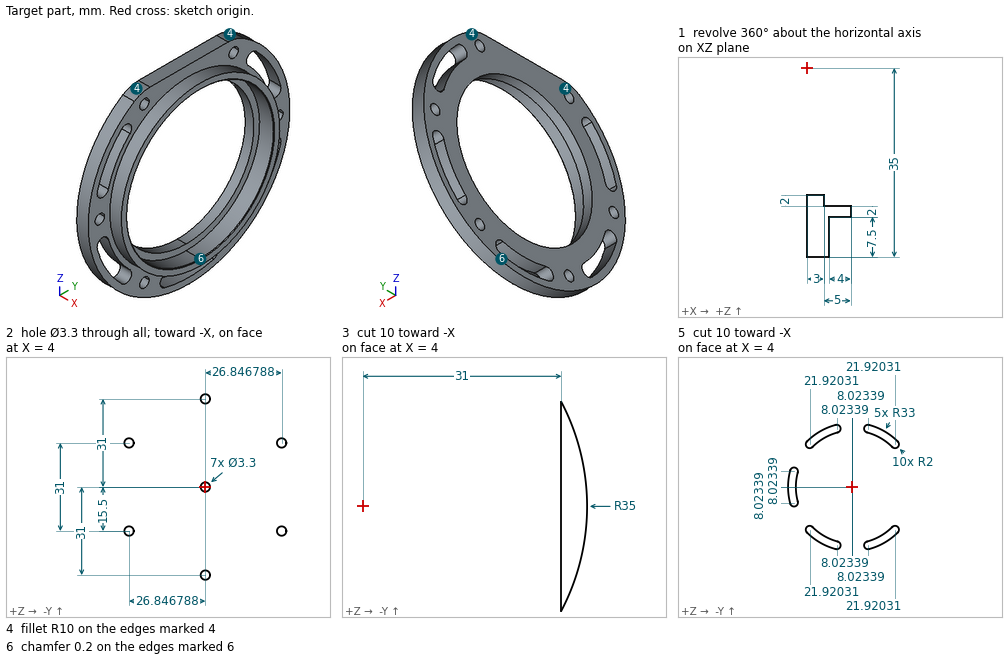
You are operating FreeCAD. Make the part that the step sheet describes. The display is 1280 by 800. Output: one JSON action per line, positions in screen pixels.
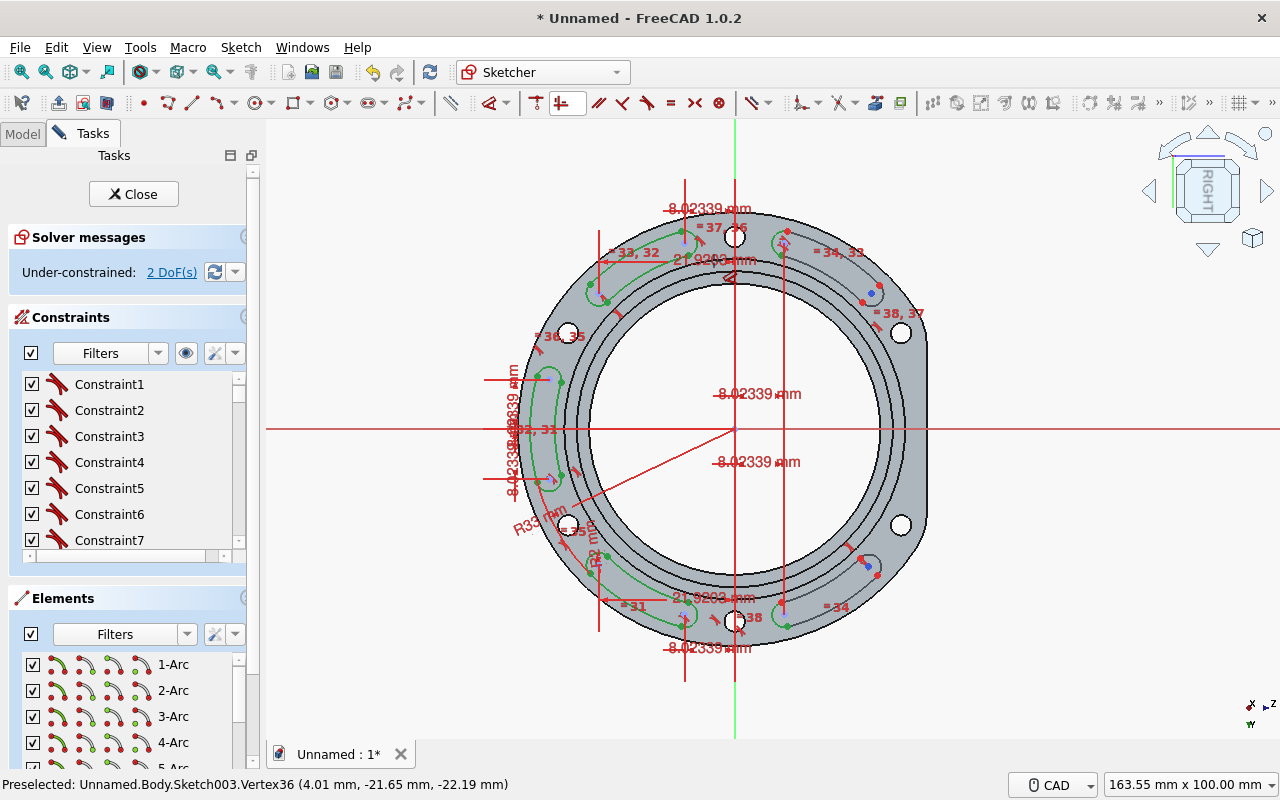
{"action": "left_click", "coordinate": [871, 294]}
{"action": "left_click", "coordinate": [834, 463]}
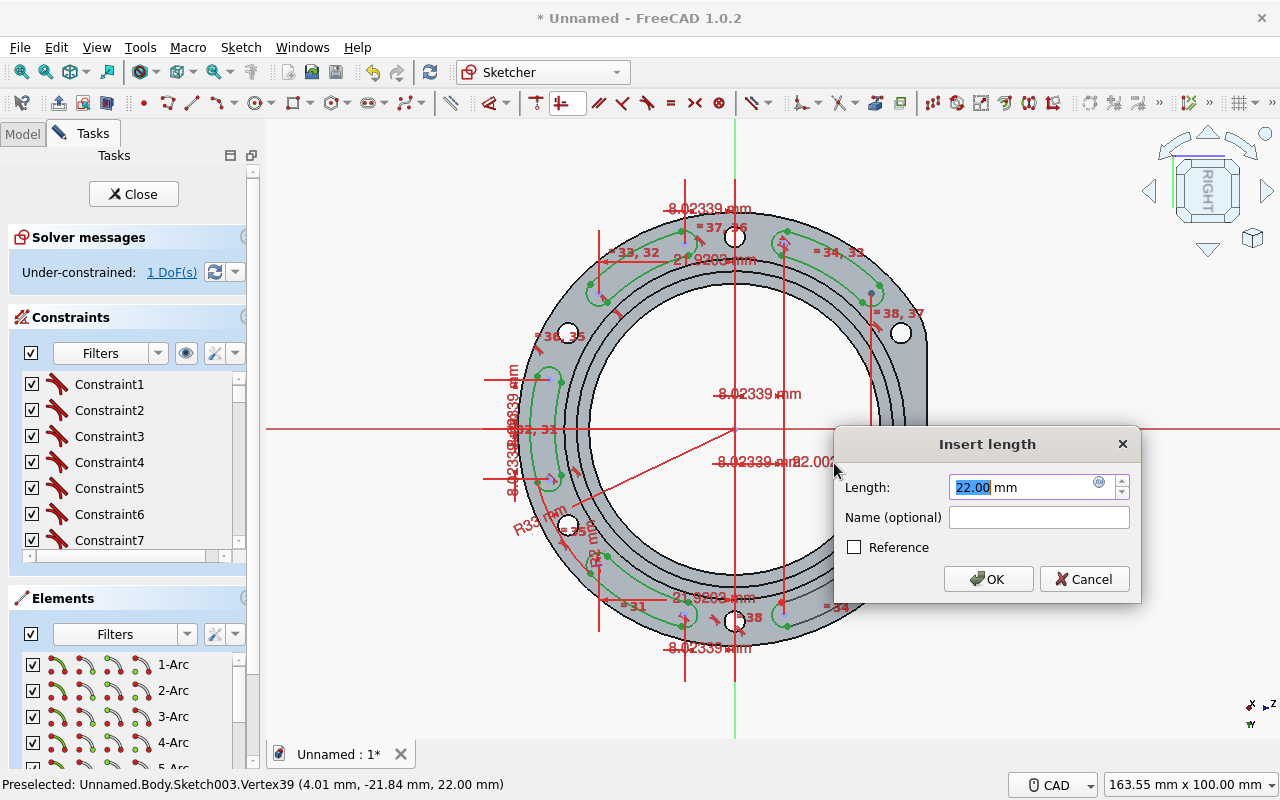
{"action": "type", "text": "21.92031"}
{"action": "key", "text": "Return"}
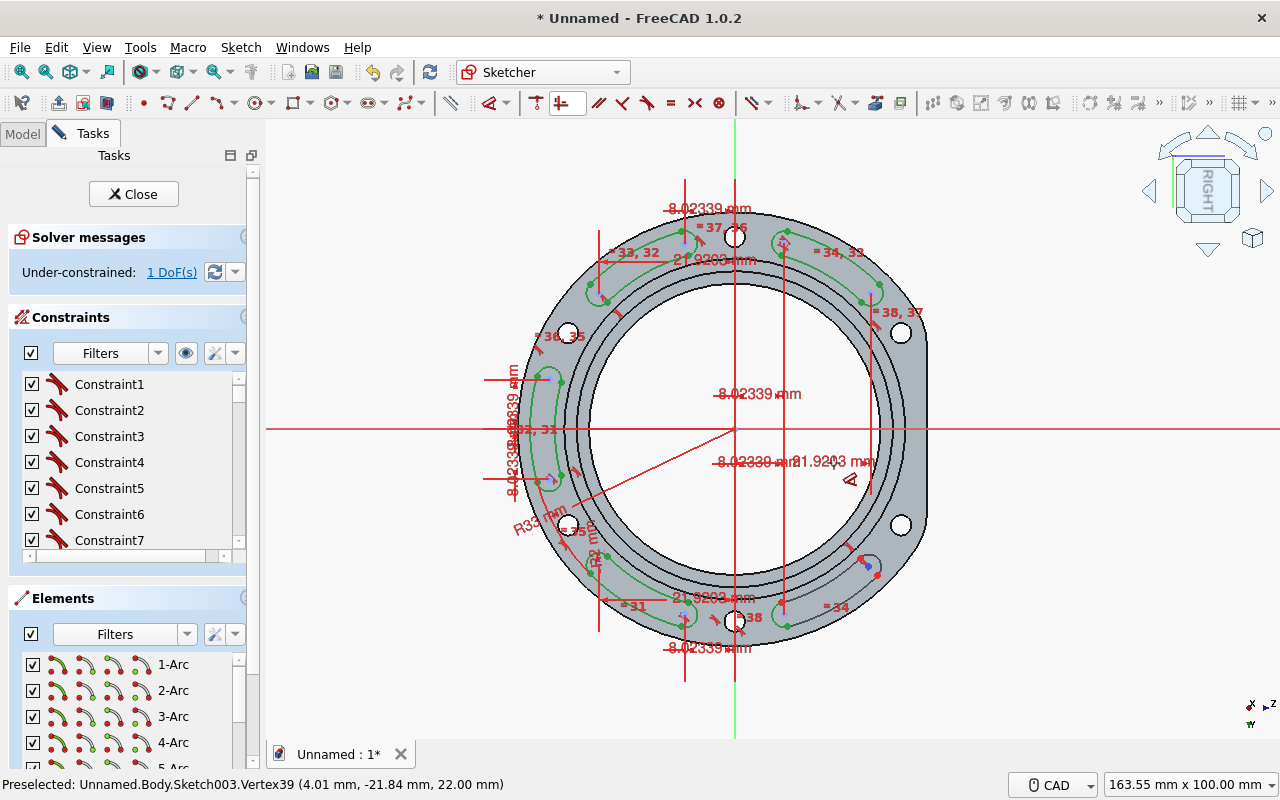
{"action": "left_click", "coordinate": [869, 567]}
{"action": "left_click", "coordinate": [833, 395]}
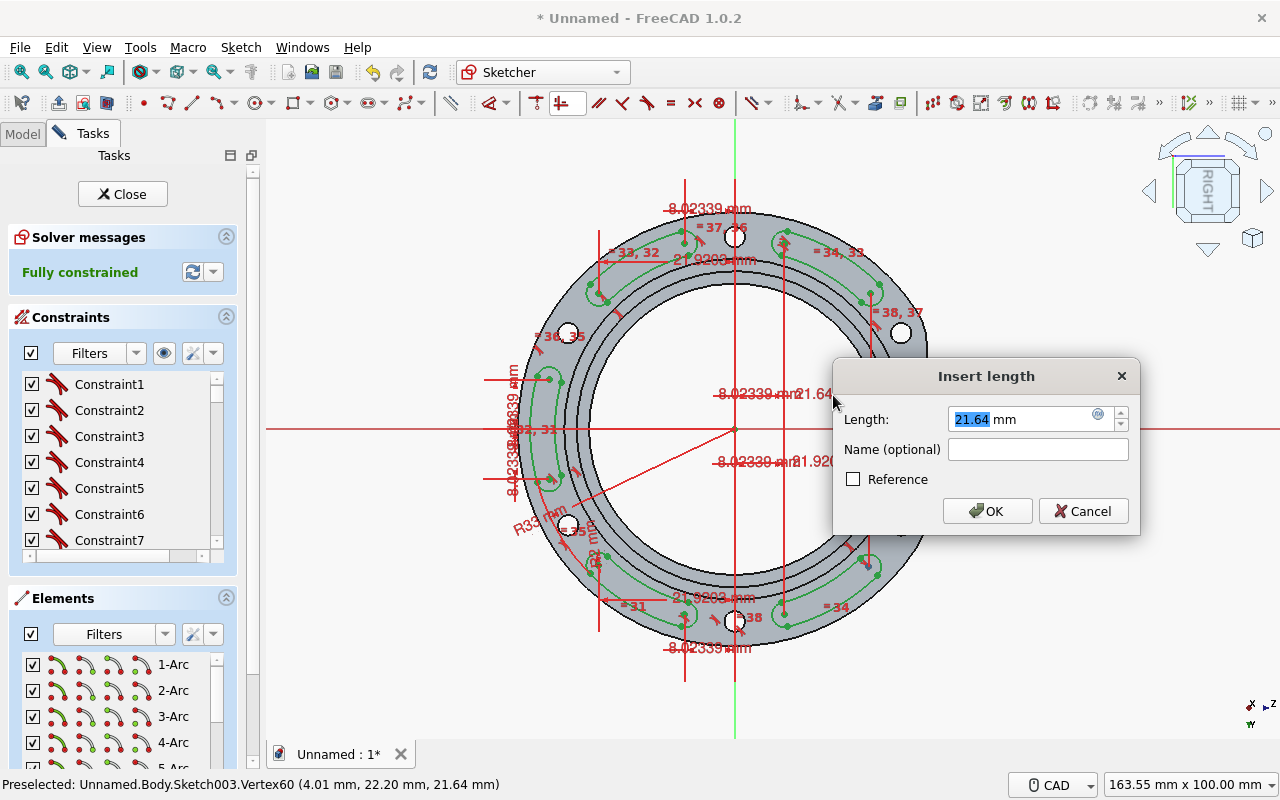
{"action": "type", "text": "21.92031"}
{"action": "key", "text": "Return"}
{"action": "key", "text": "Escape"}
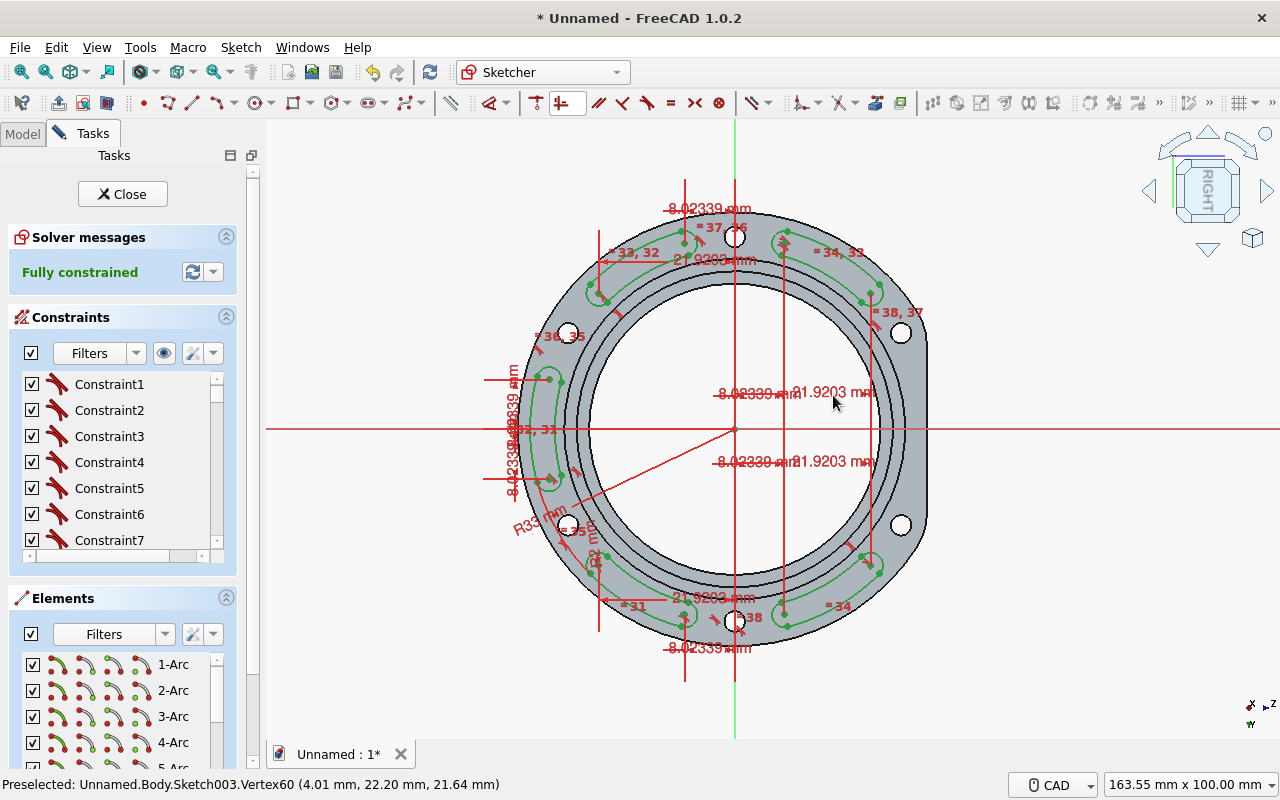
{"action": "left_click", "coordinate": [123, 194]}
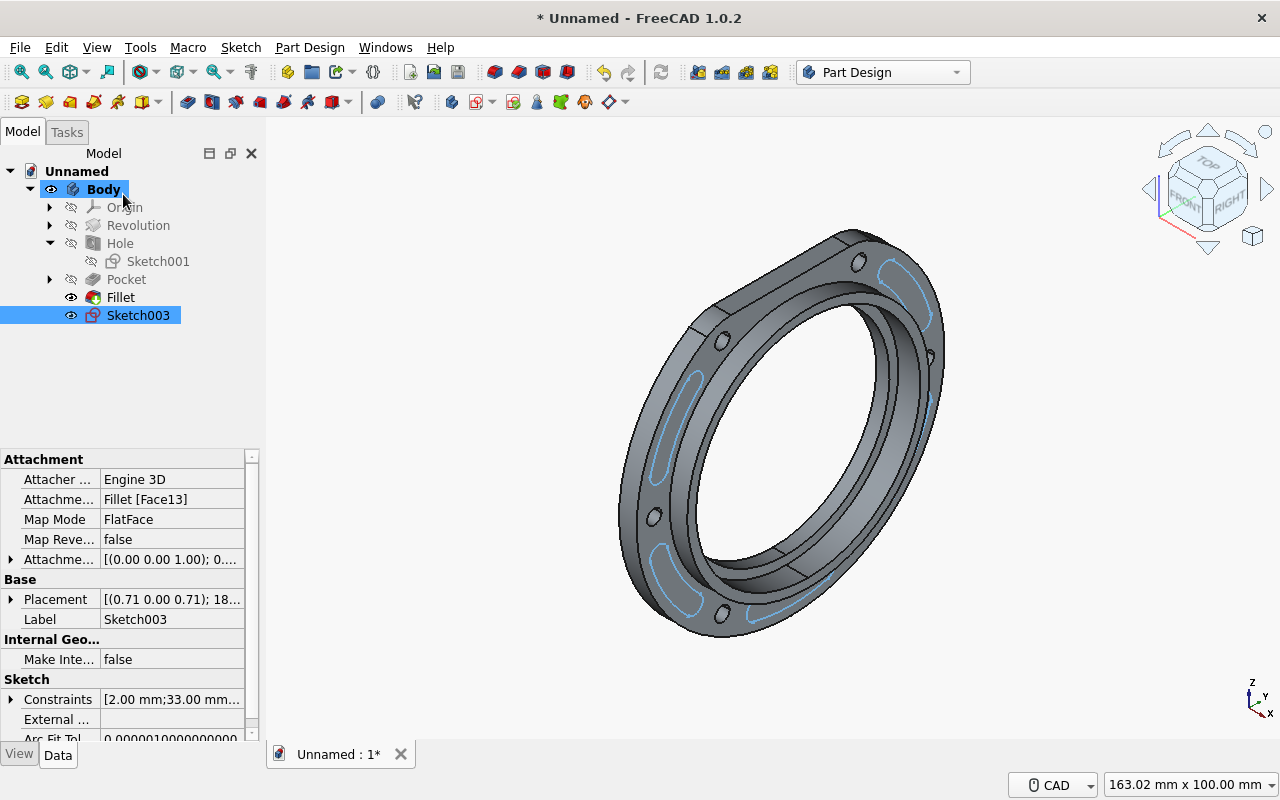
{"action": "left_click", "coordinate": [188, 102]}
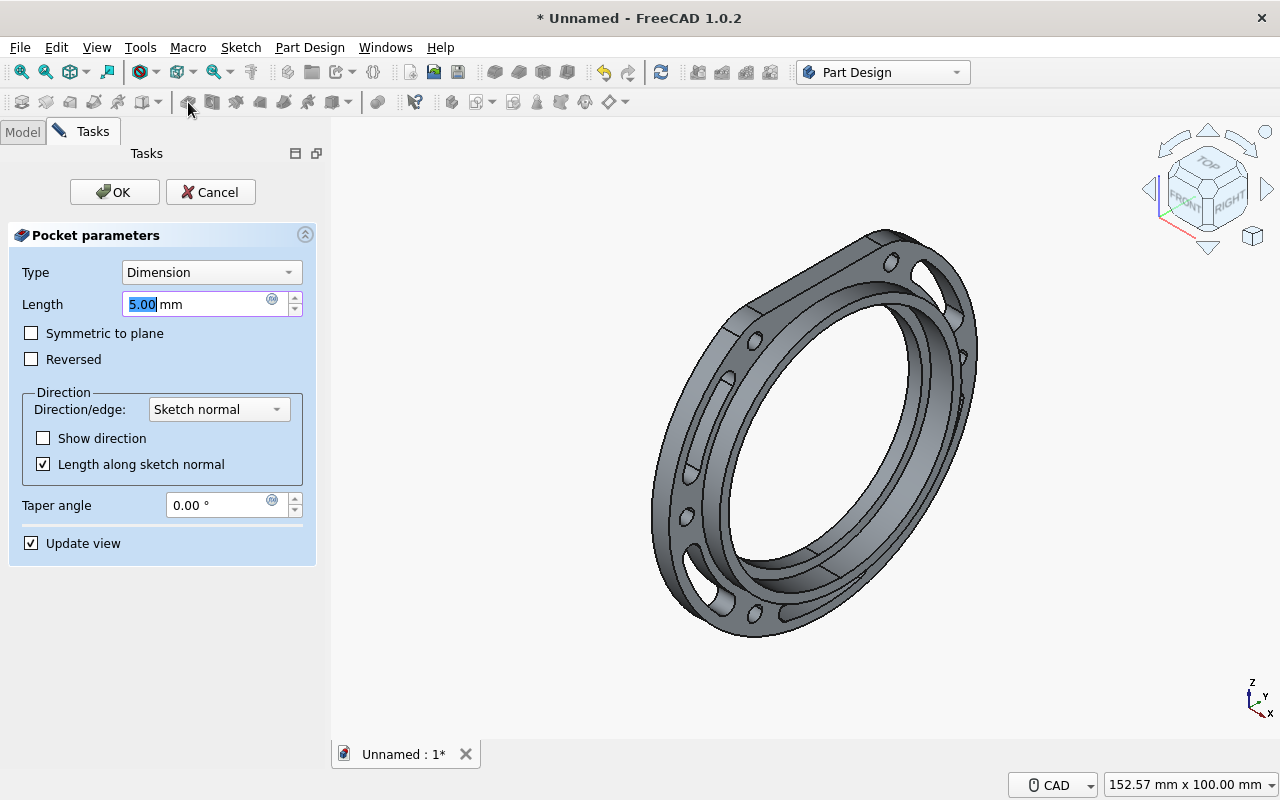
{"action": "type", "text": "10"}
{"action": "key", "text": "Tab"}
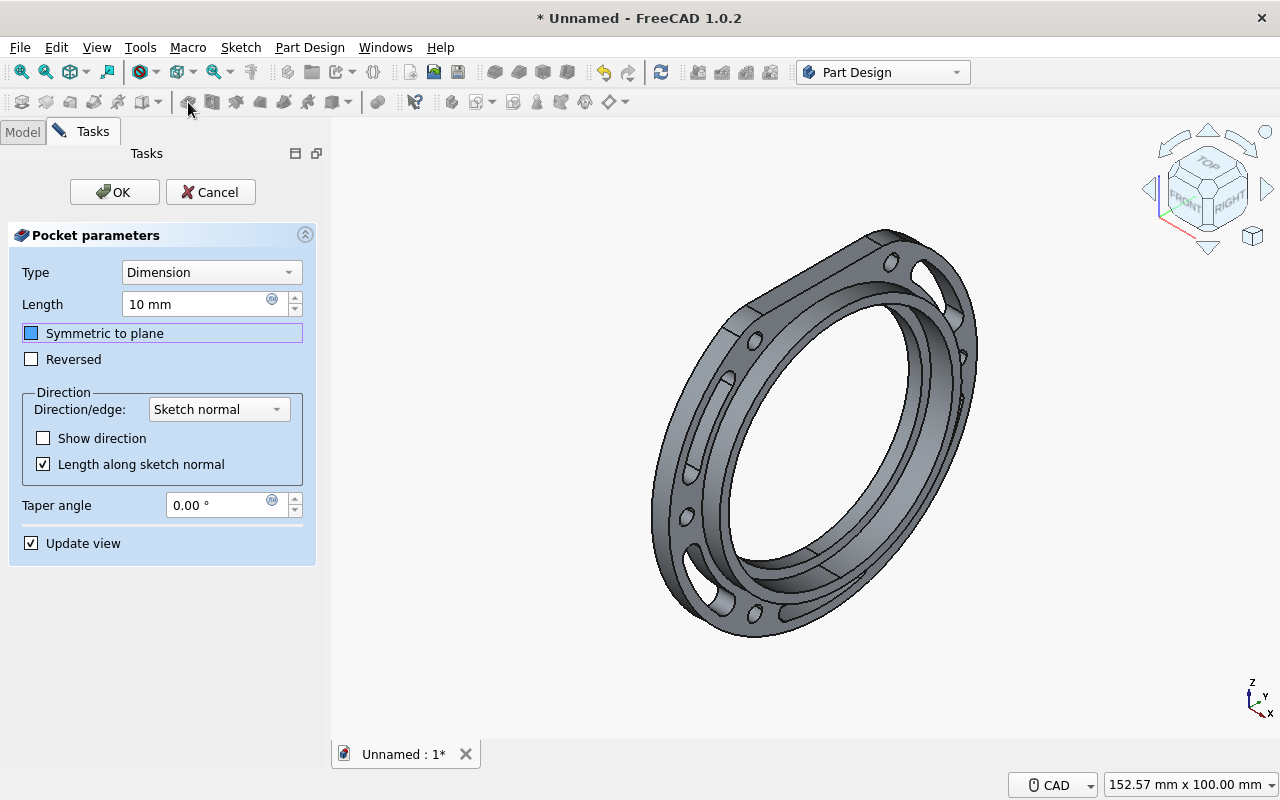
{"action": "left_click", "coordinate": [115, 192]}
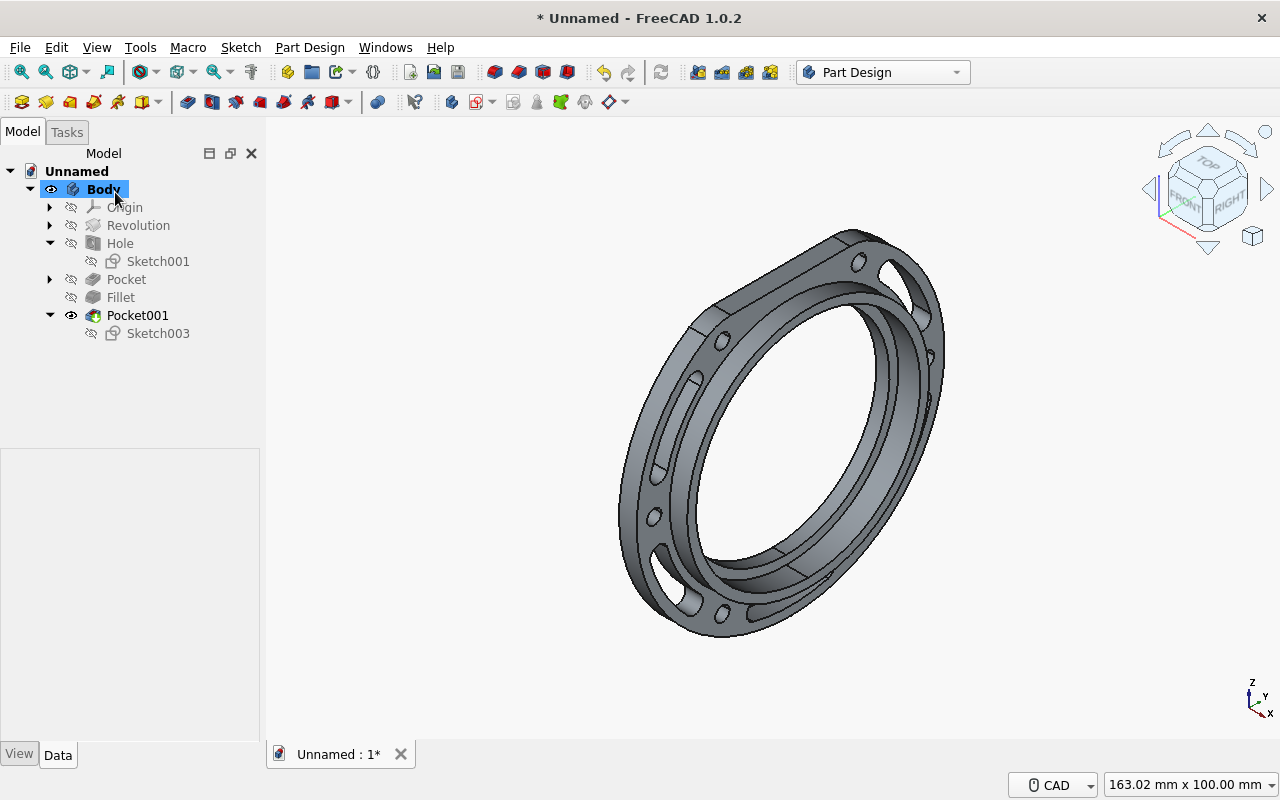
{"action": "left_click", "coordinate": [915, 346]}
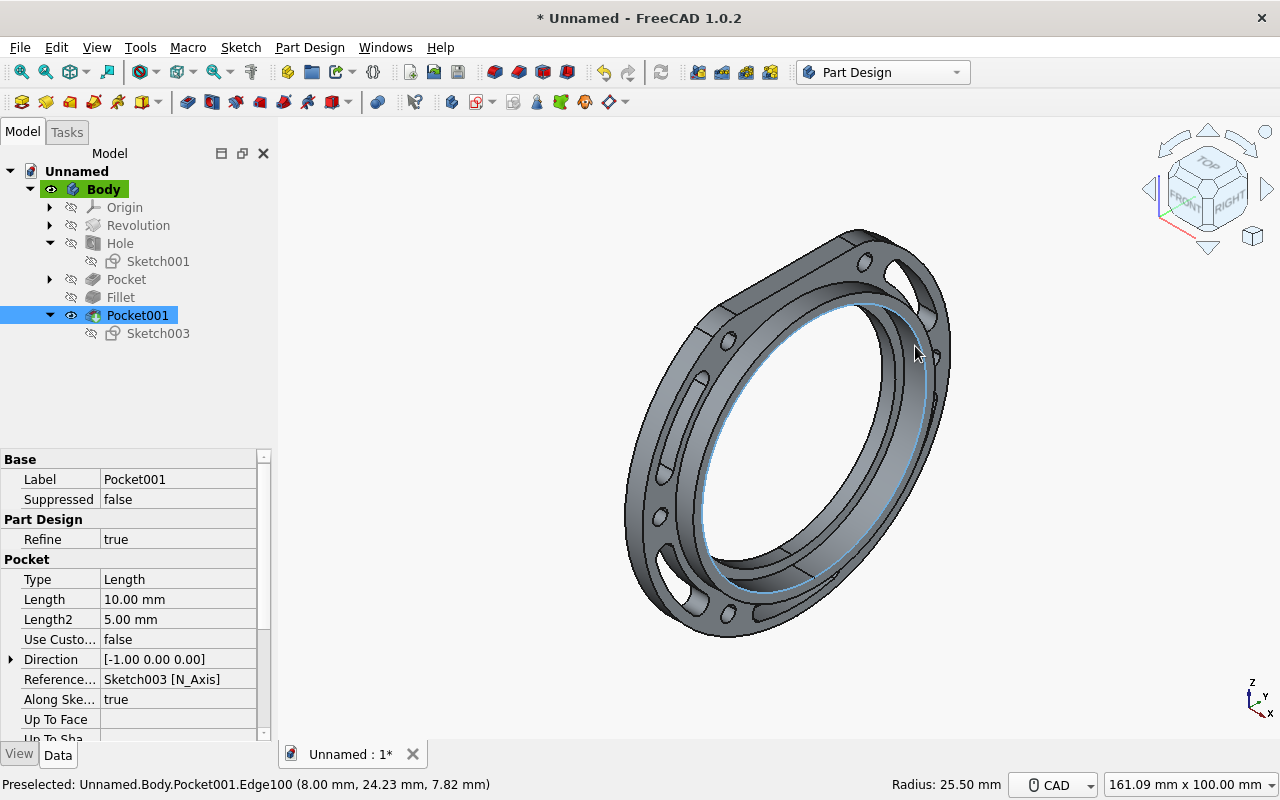
{"action": "left_click", "coordinate": [520, 72]}